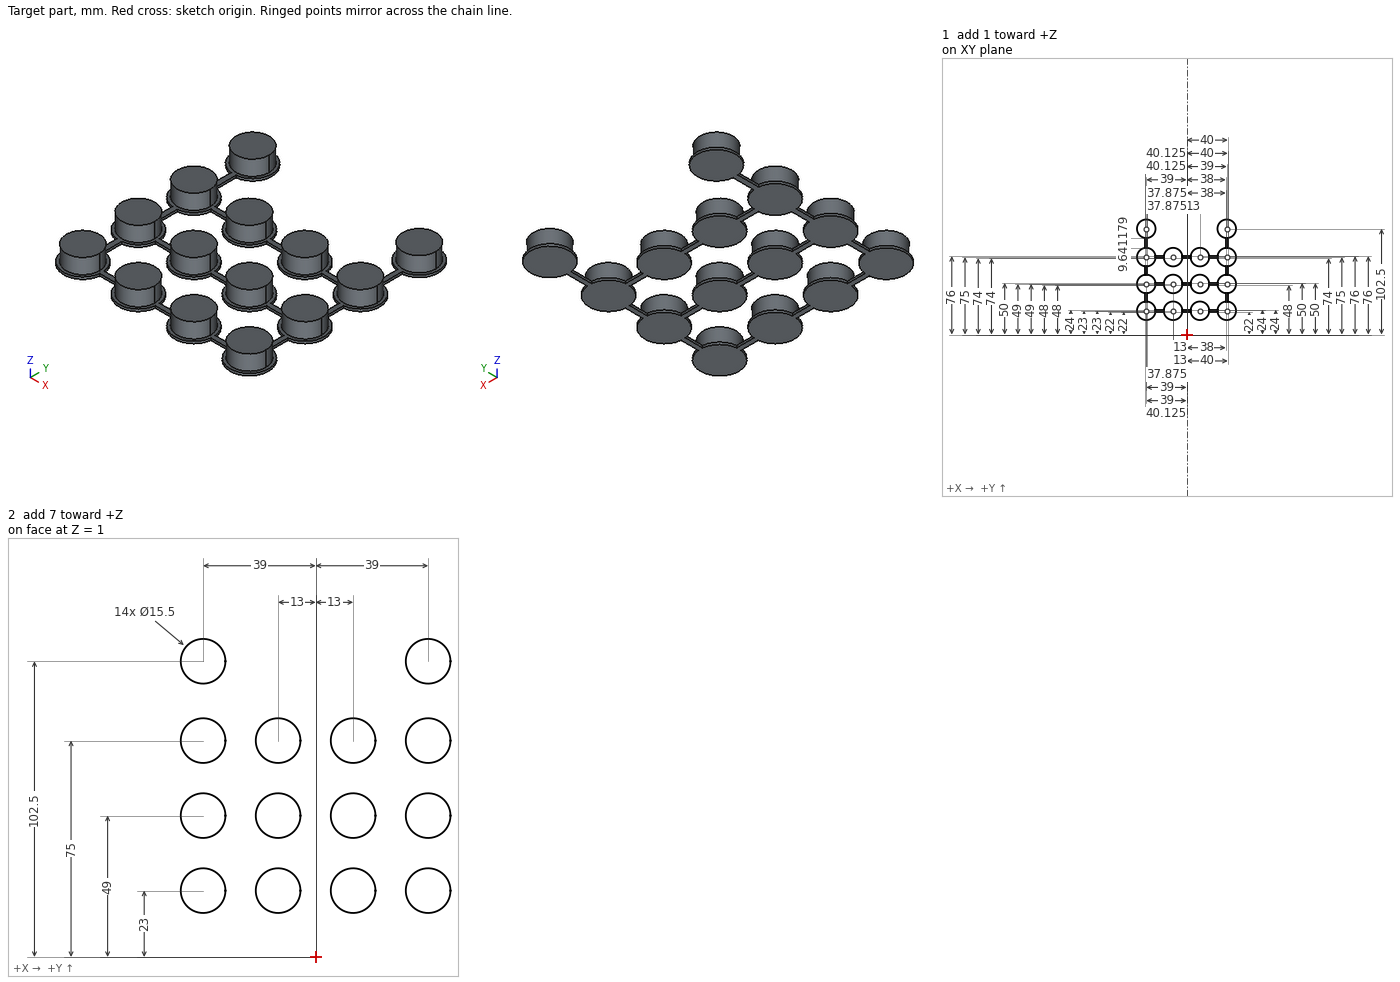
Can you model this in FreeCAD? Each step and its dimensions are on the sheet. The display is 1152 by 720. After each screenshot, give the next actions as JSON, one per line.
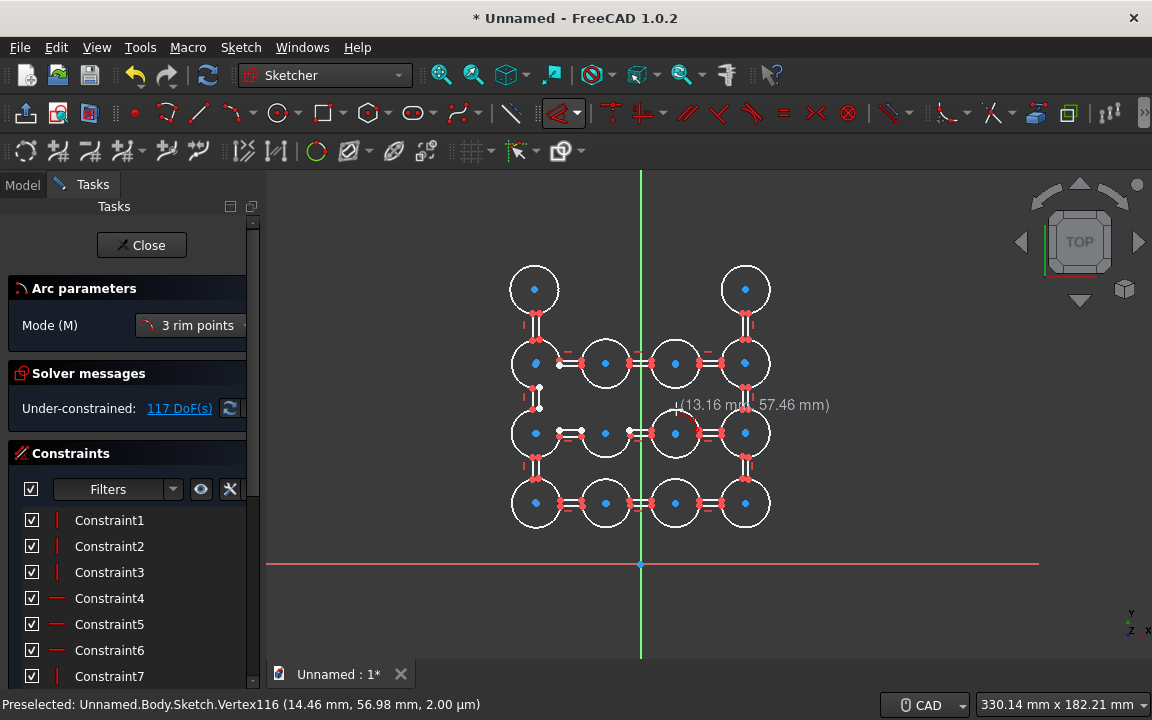
{"action": "scroll", "coordinate": [630, 430], "scroll_direction": "up", "scroll_amount": 6}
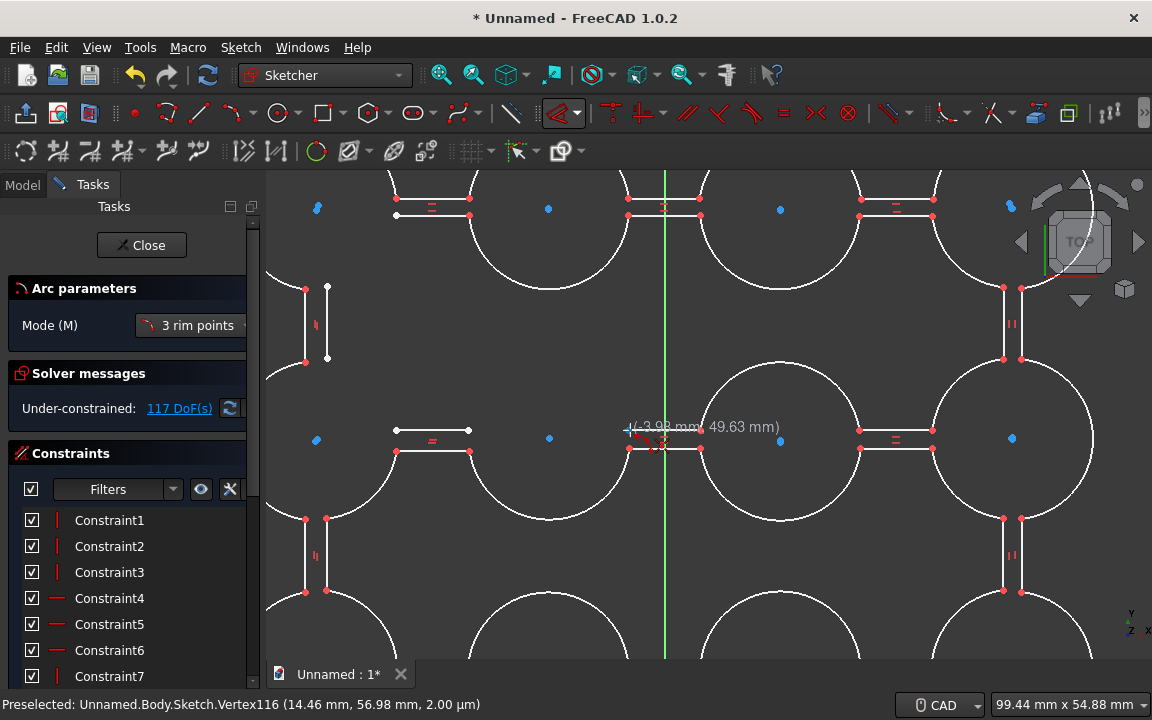
{"action": "left_click", "coordinate": [629, 430]}
{"action": "left_click", "coordinate": [469, 430]}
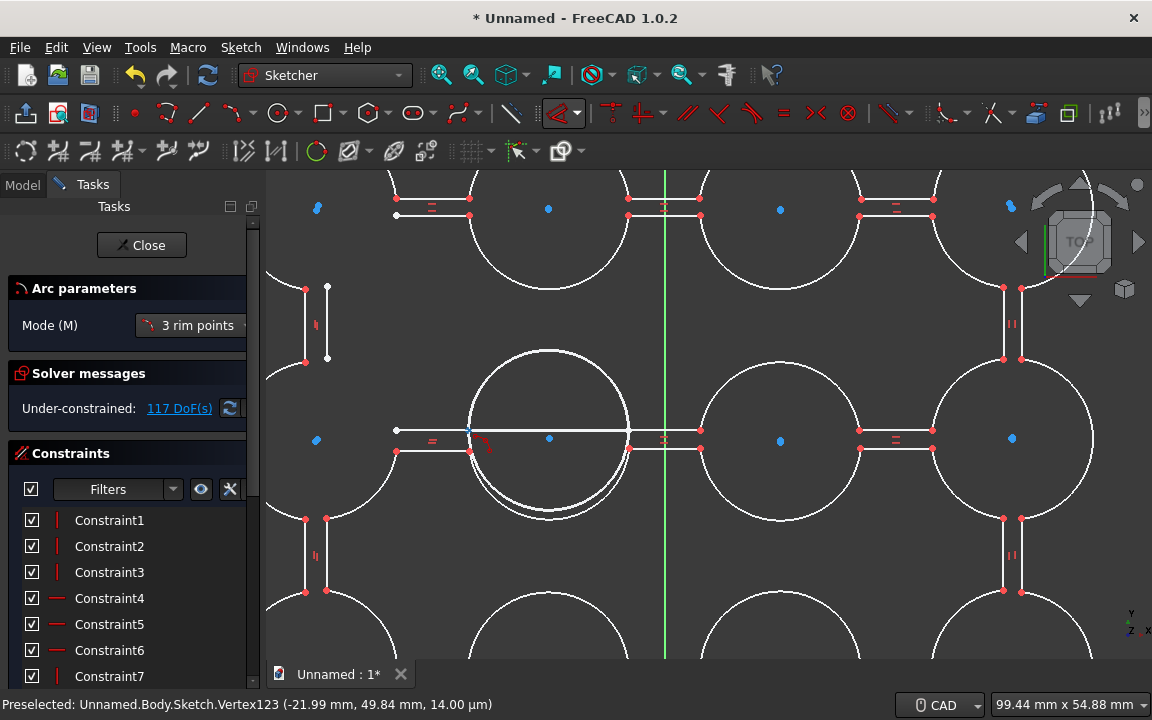
{"action": "scroll", "coordinate": [630, 430], "scroll_direction": "down", "scroll_amount": 6}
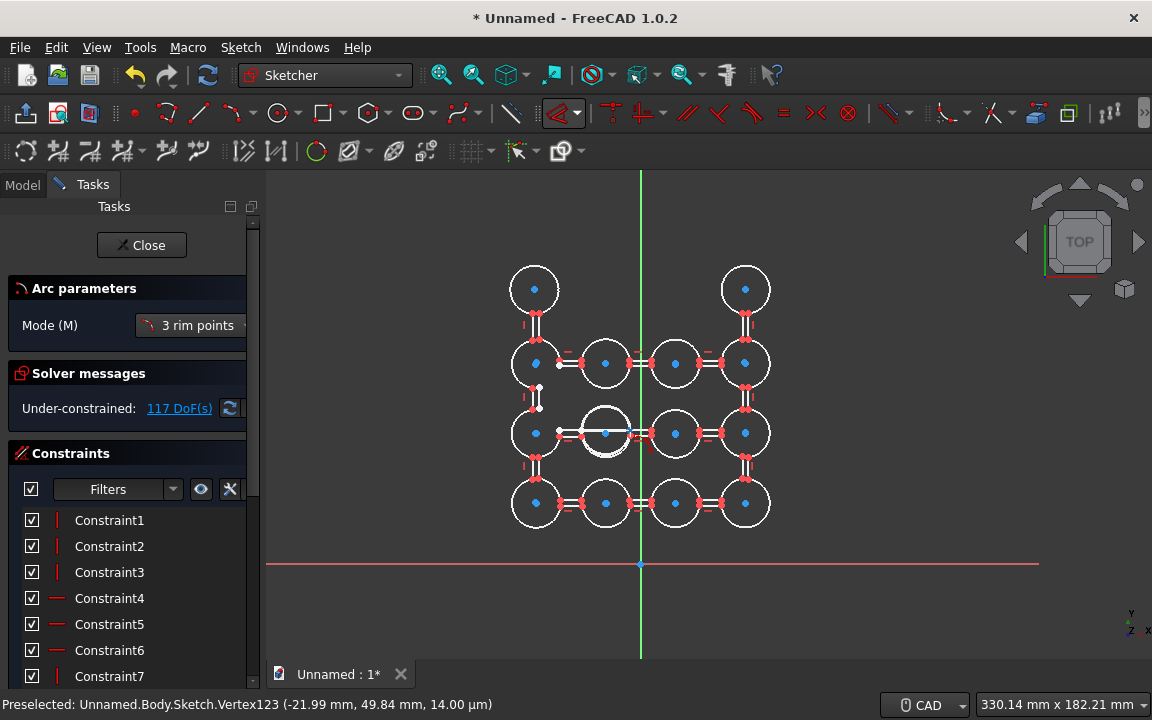
{"action": "left_click", "coordinate": [606, 409]}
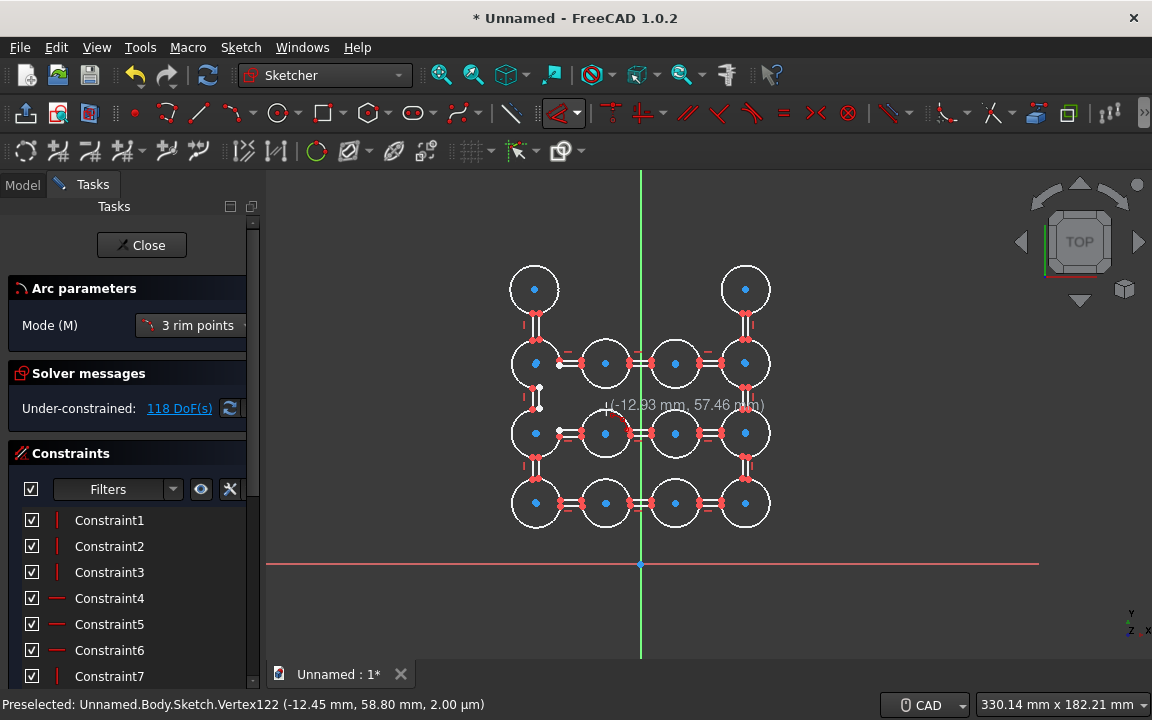
{"action": "scroll", "coordinate": [560, 430], "scroll_direction": "up", "scroll_amount": 6}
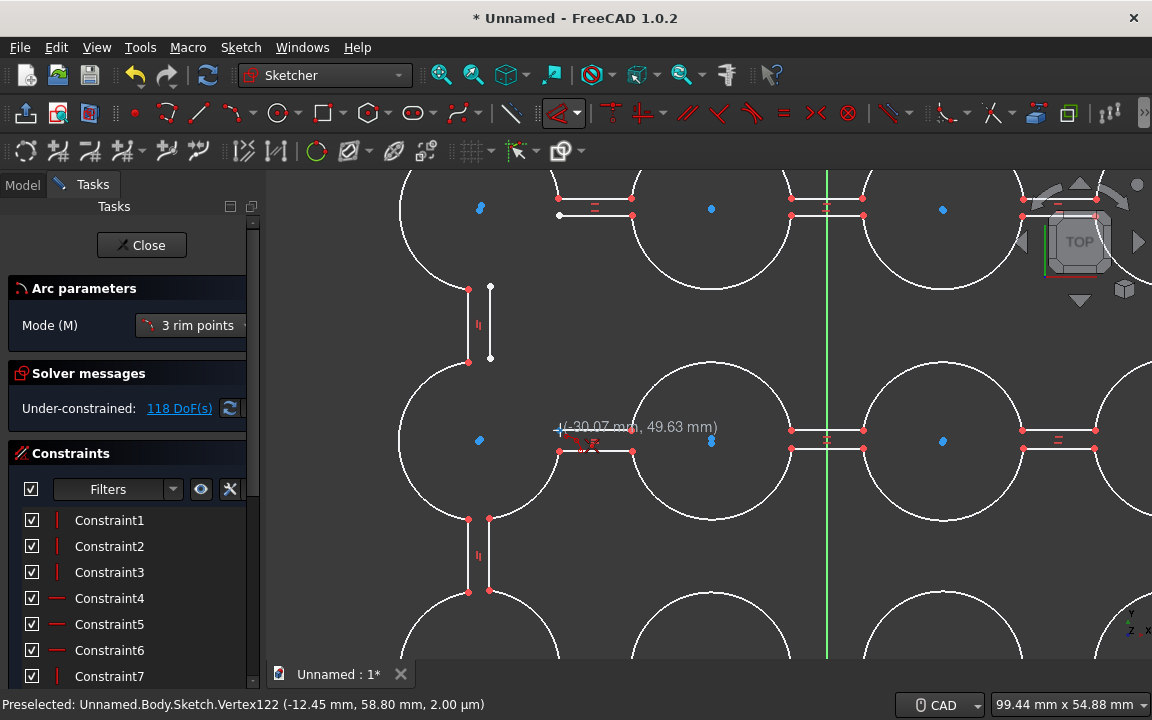
{"action": "left_click", "coordinate": [559, 430]}
{"action": "left_click", "coordinate": [490, 359]}
{"action": "left_click", "coordinate": [537, 381]}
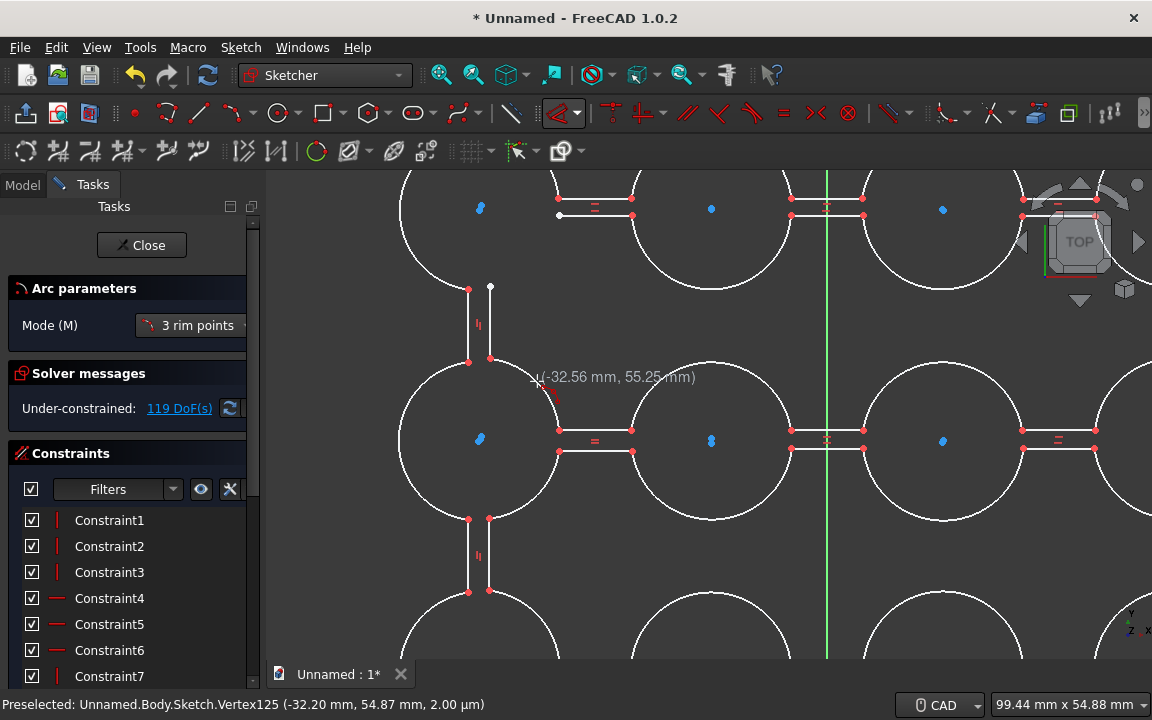
{"action": "left_click", "coordinate": [490, 287]}
{"action": "left_click", "coordinate": [559, 216]}
{"action": "left_click", "coordinate": [537, 262]}
{"action": "key", "text": "Escape"}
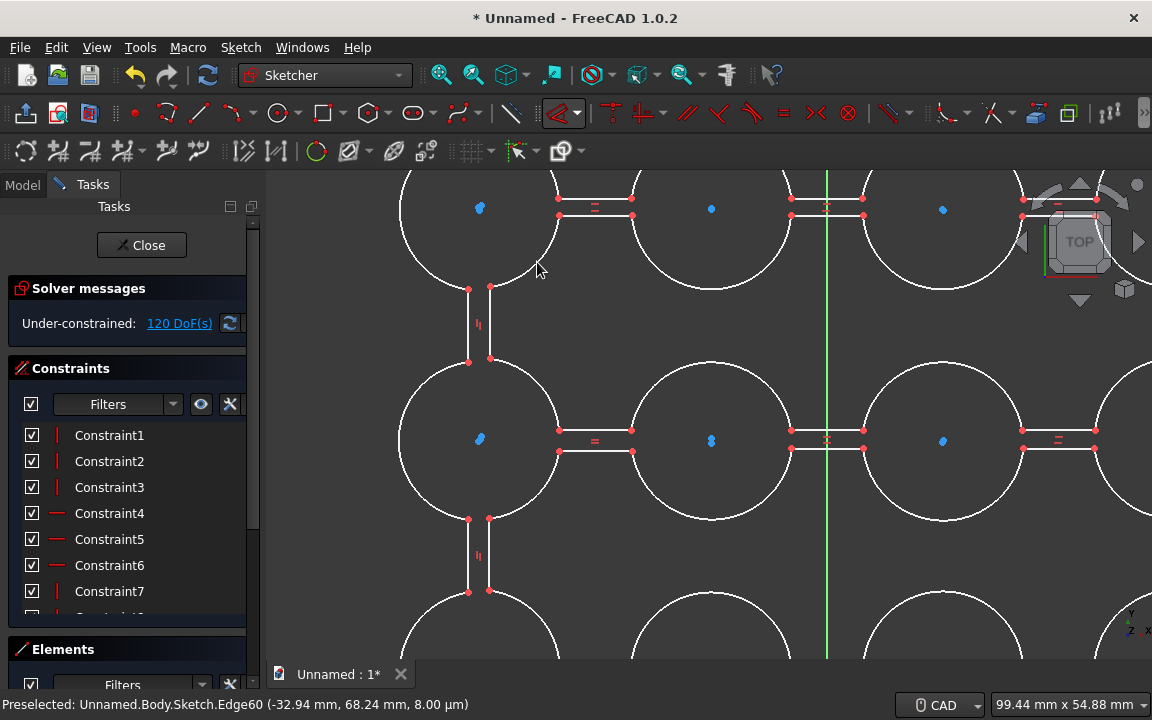
{"action": "scroll", "coordinate": [560, 430], "scroll_direction": "down", "scroll_amount": 6}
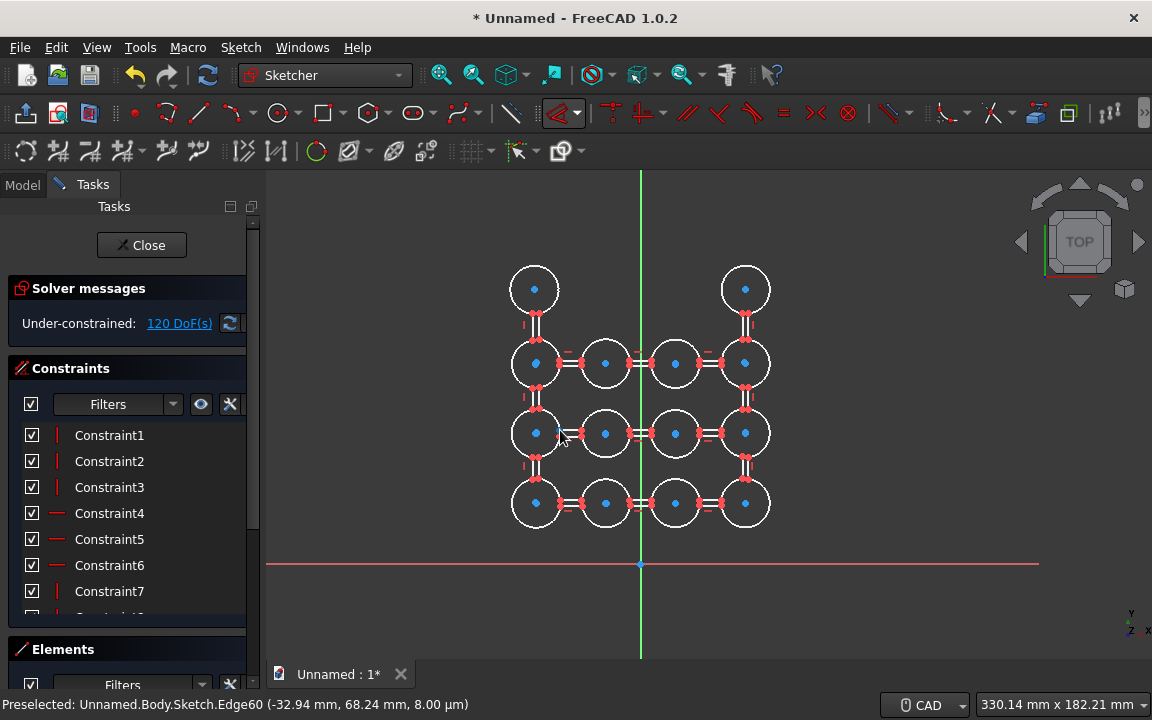
{"action": "left_click", "coordinate": [766, 377]}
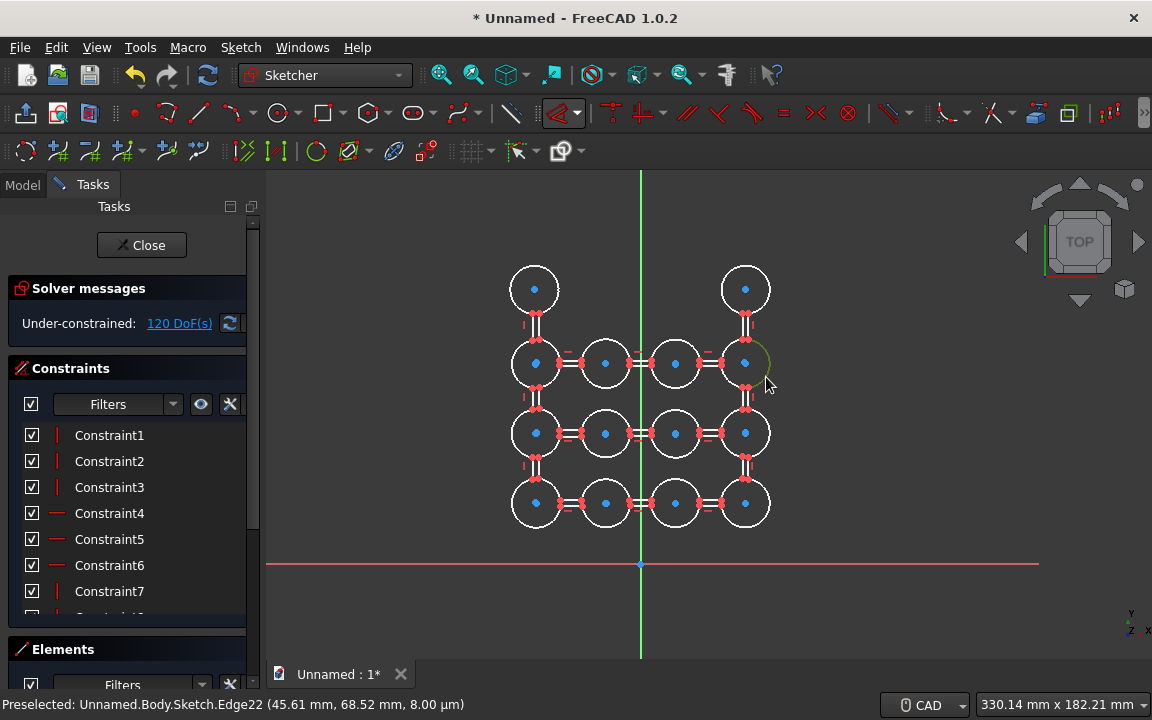
{"action": "scroll", "coordinate": [733, 342], "scroll_direction": "up", "scroll_amount": 2}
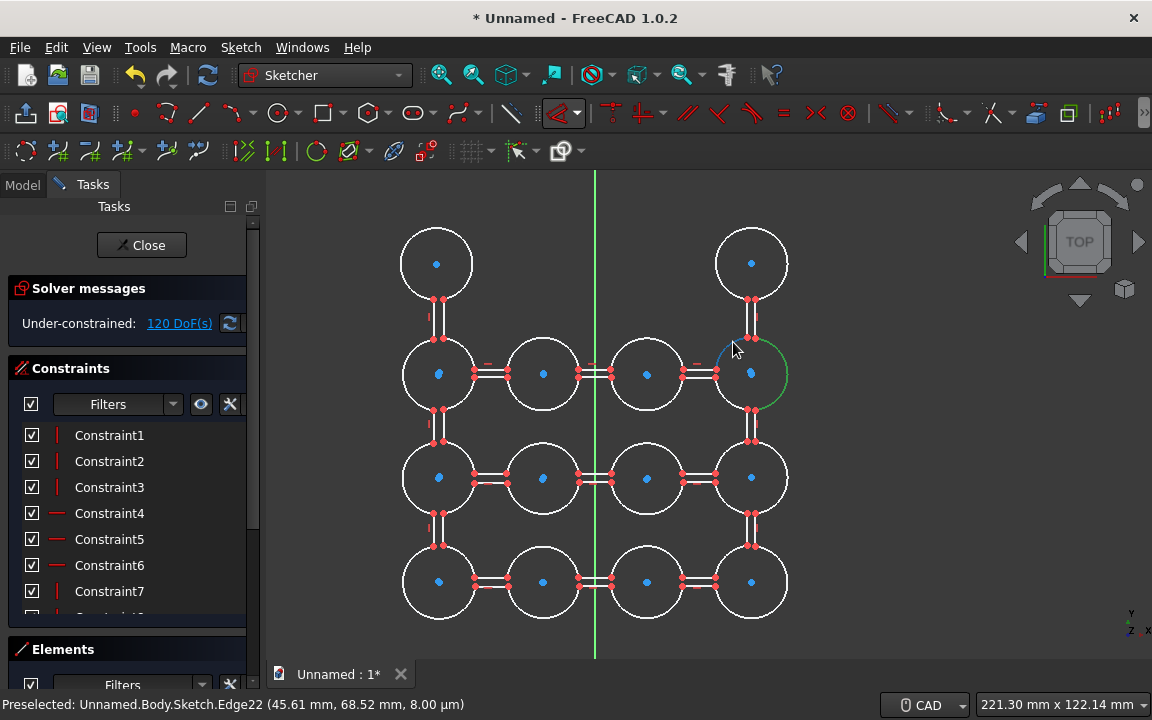
{"action": "left_click", "coordinate": [733, 342]}